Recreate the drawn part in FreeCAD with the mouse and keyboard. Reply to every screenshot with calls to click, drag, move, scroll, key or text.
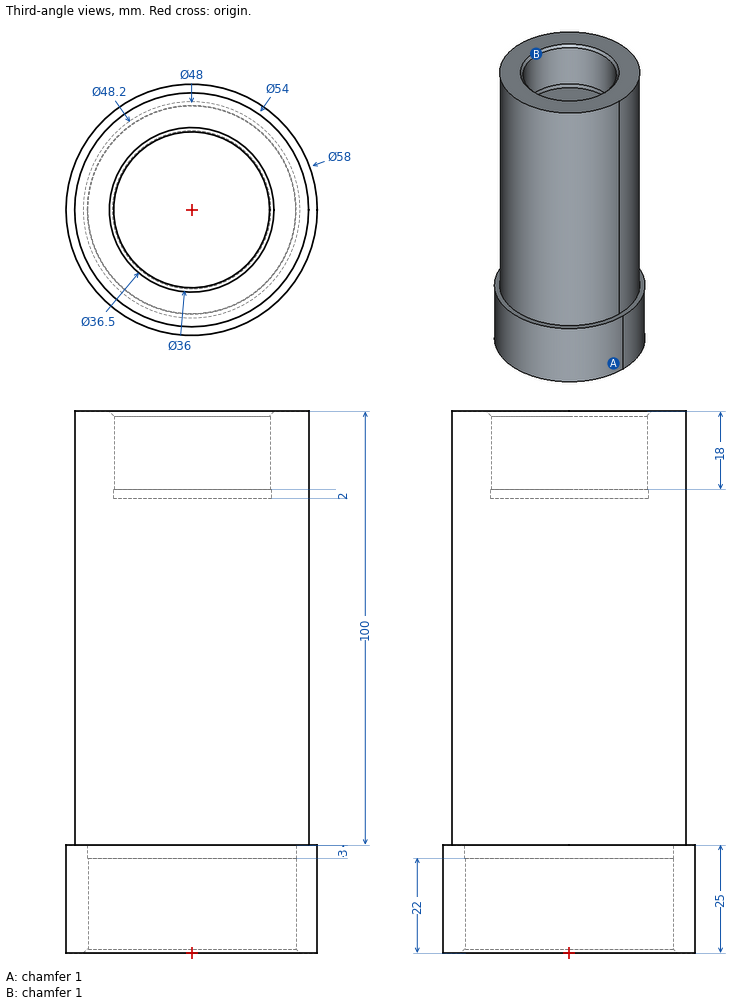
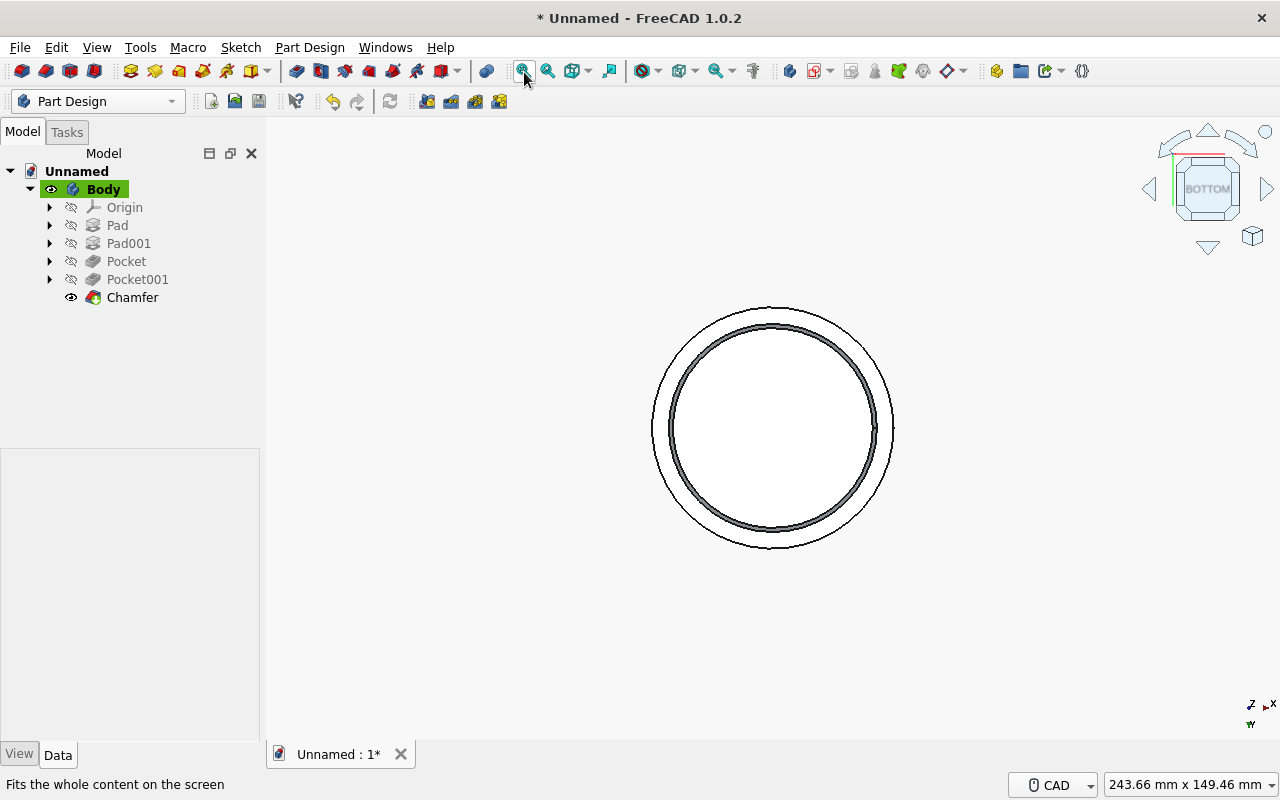
key(0)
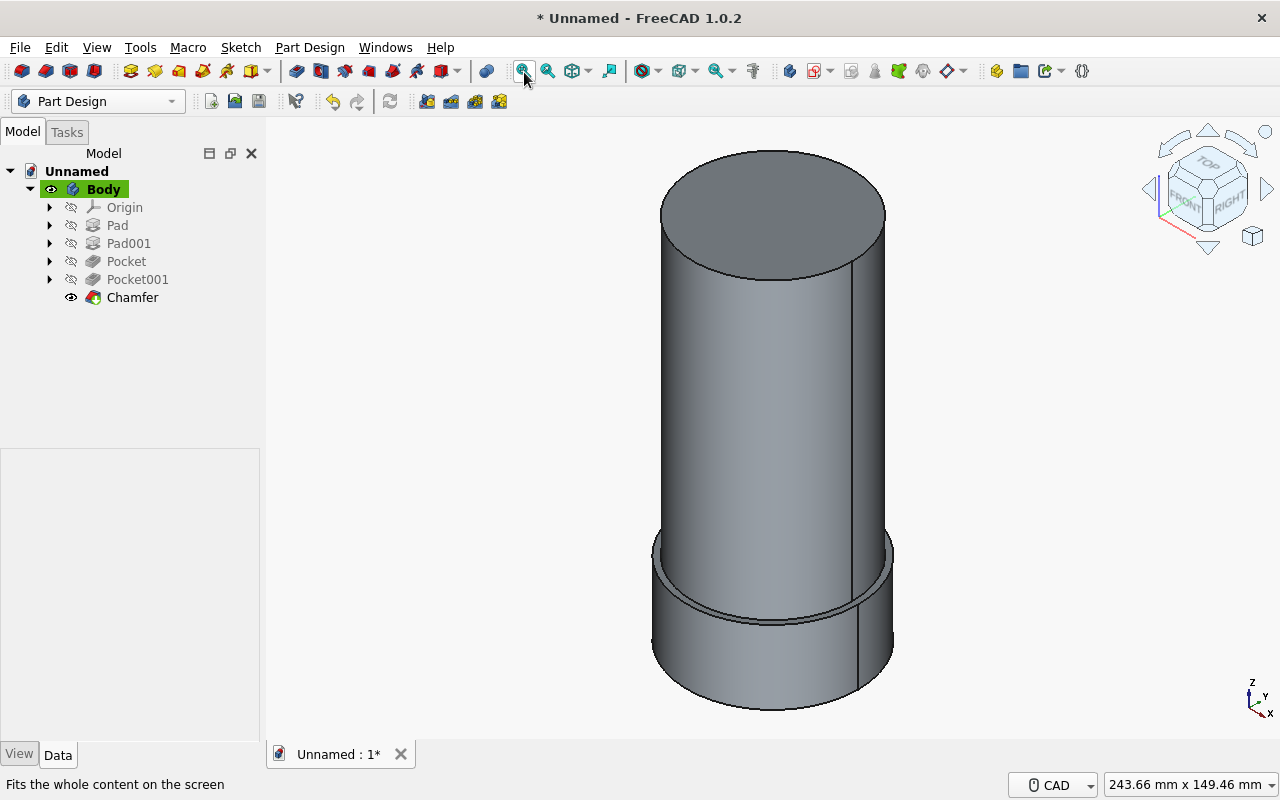
click(524, 72)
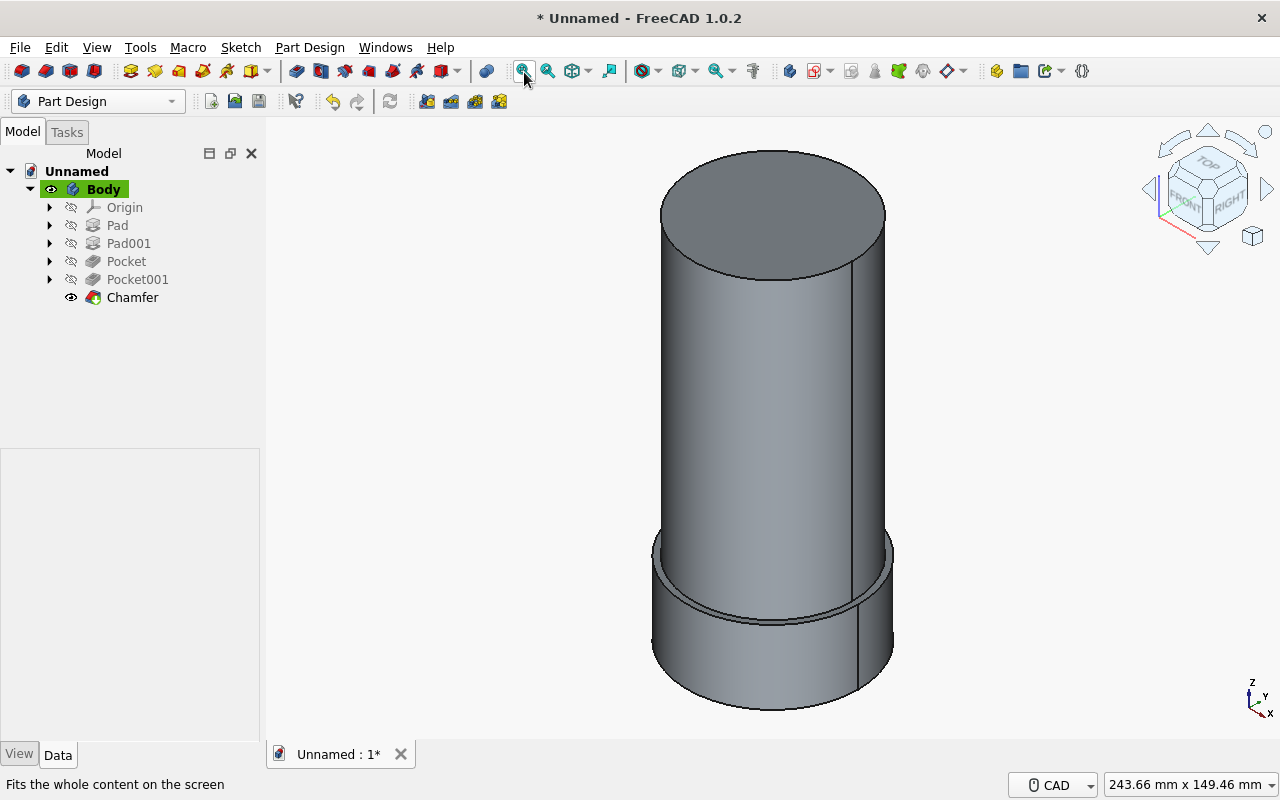
click(773, 215)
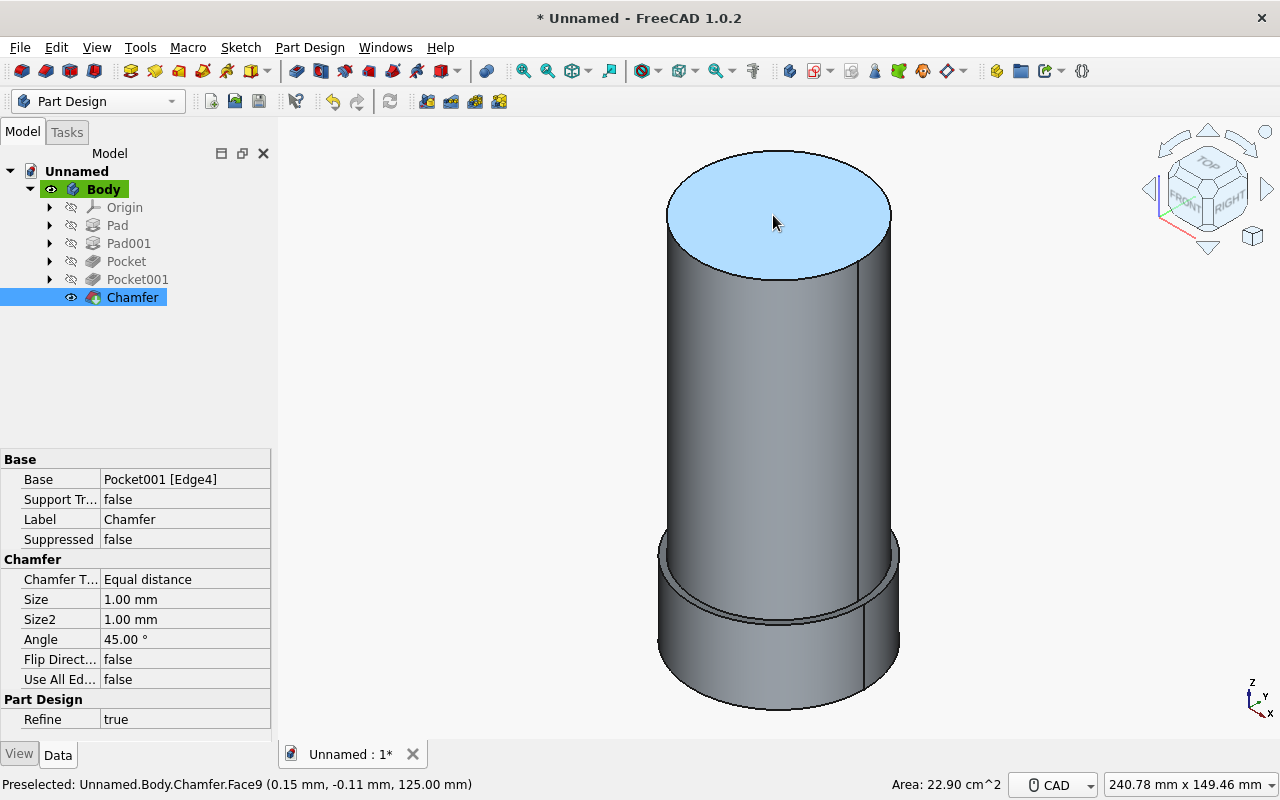
click(814, 72)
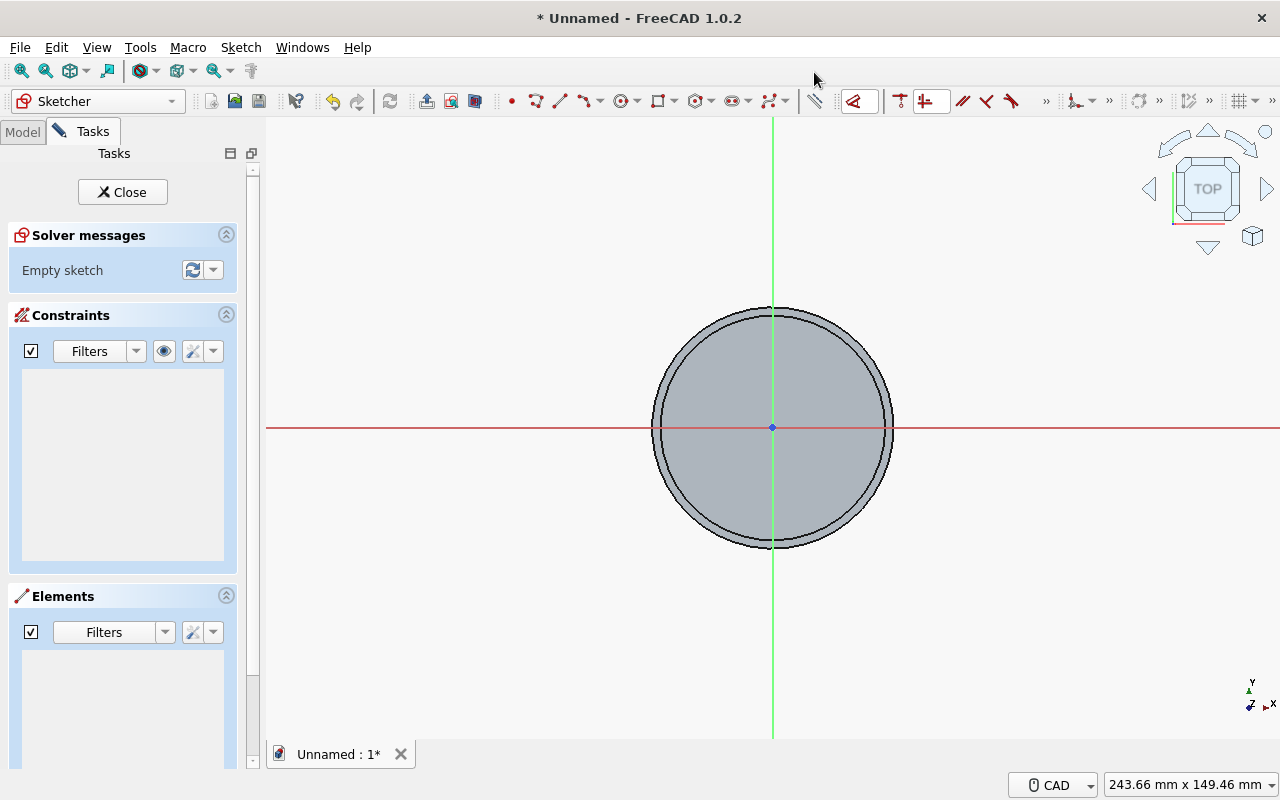
scroll(813, 428, up, 5)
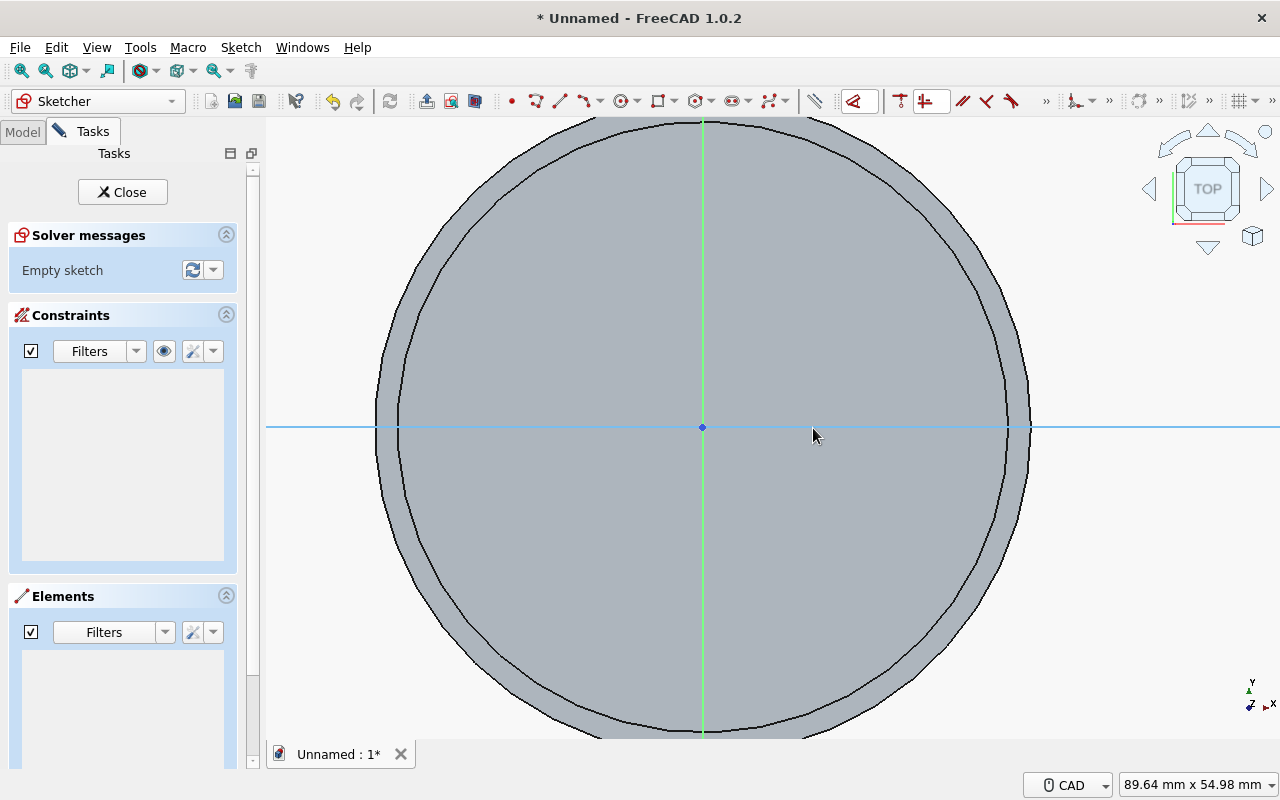
click(622, 102)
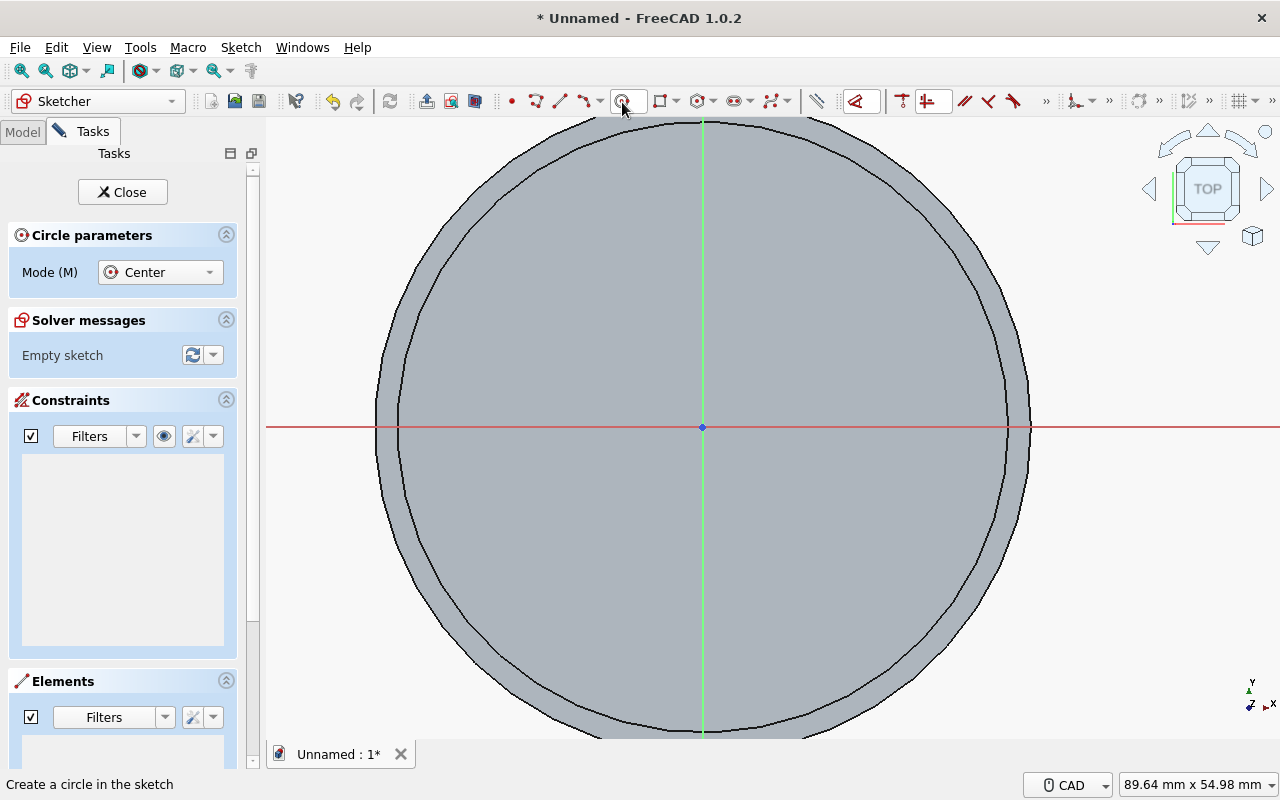
click(703, 427)
move(847, 283)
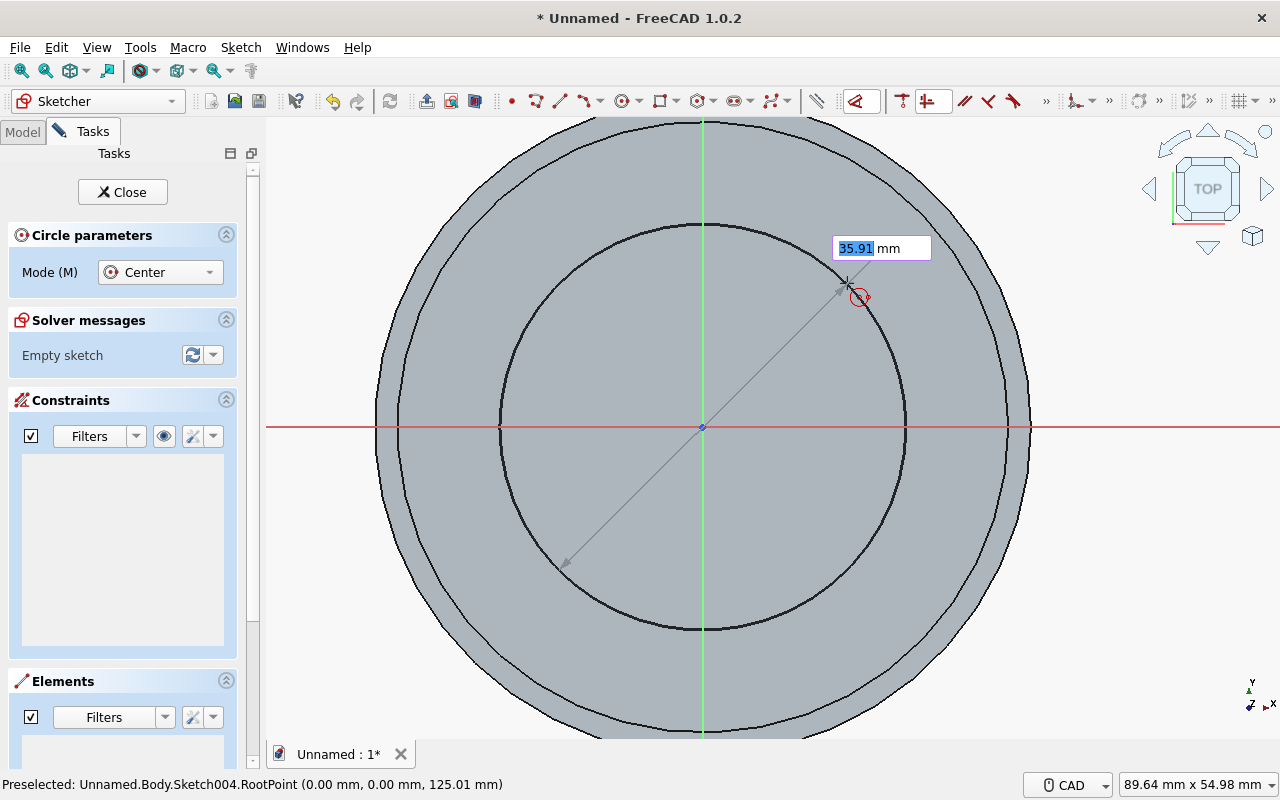
text(36)
key(Return)
key(Escape)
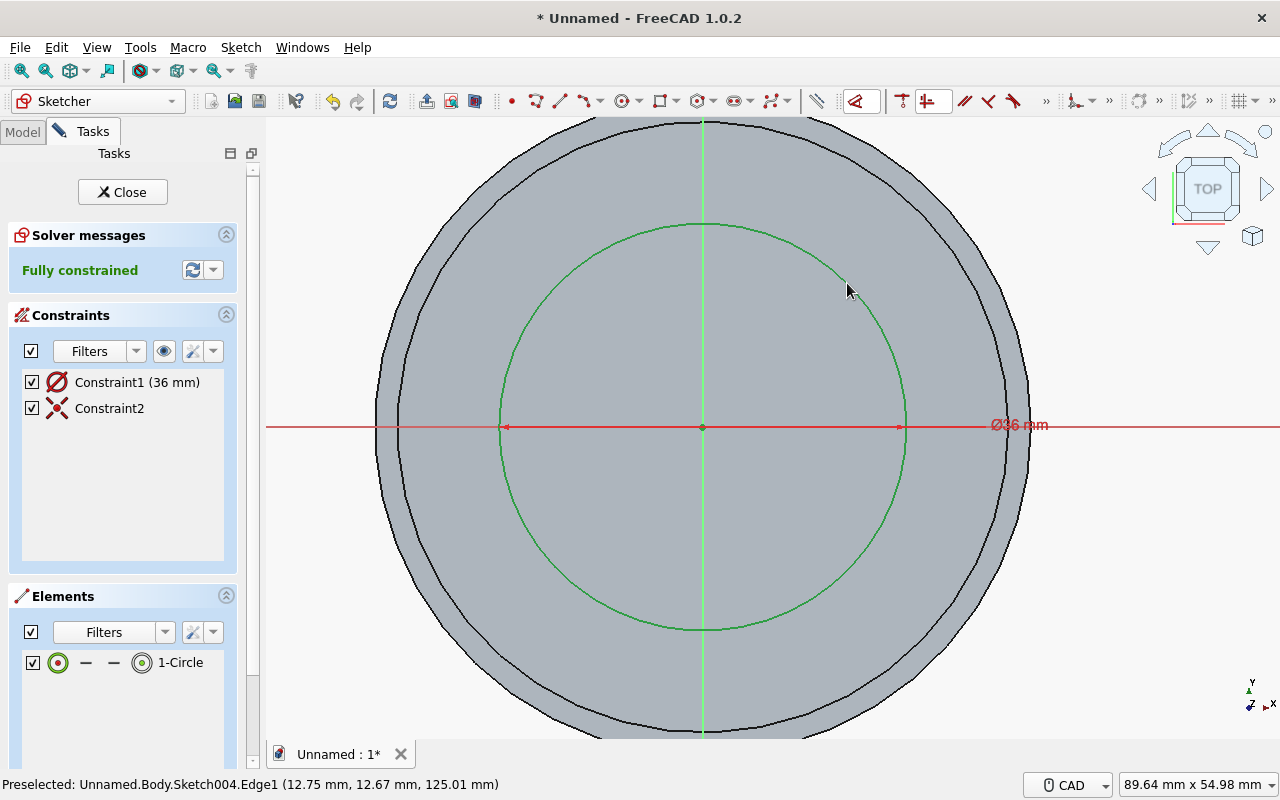
click(123, 192)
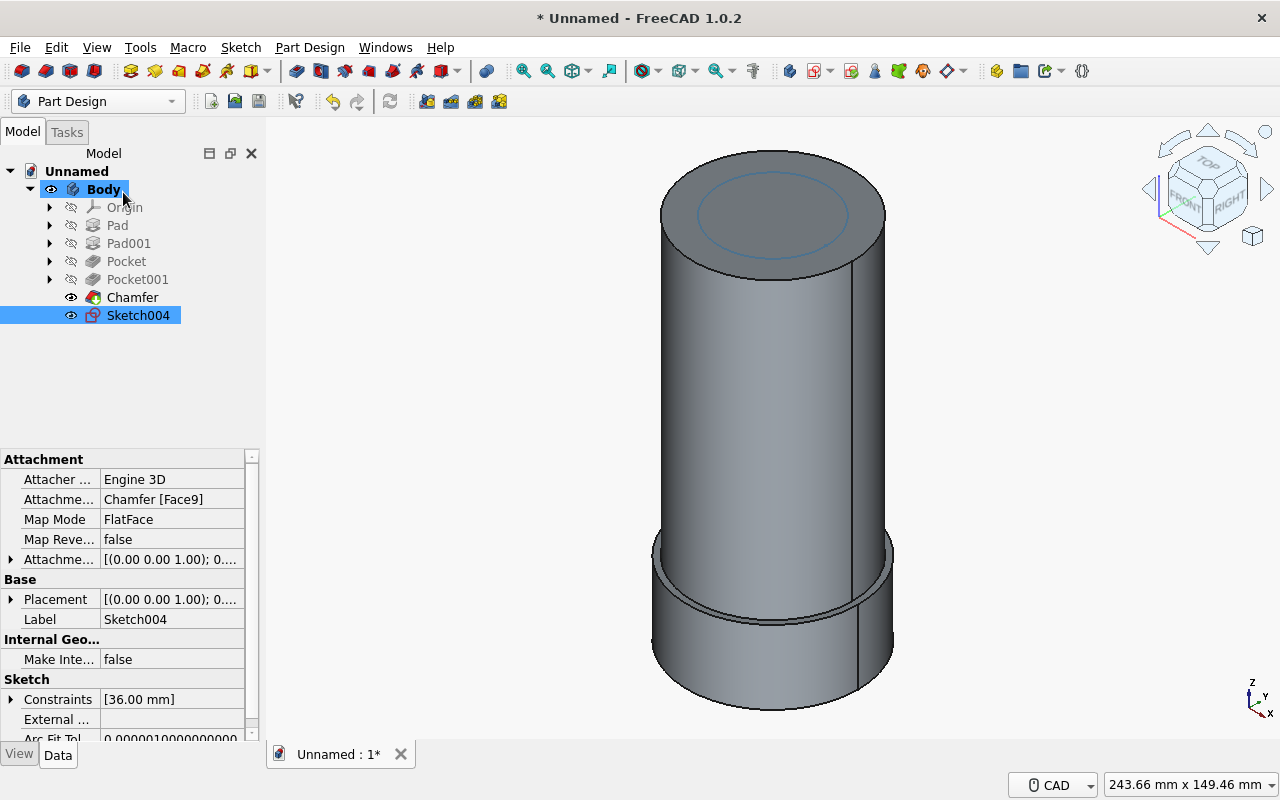
click(298, 72)